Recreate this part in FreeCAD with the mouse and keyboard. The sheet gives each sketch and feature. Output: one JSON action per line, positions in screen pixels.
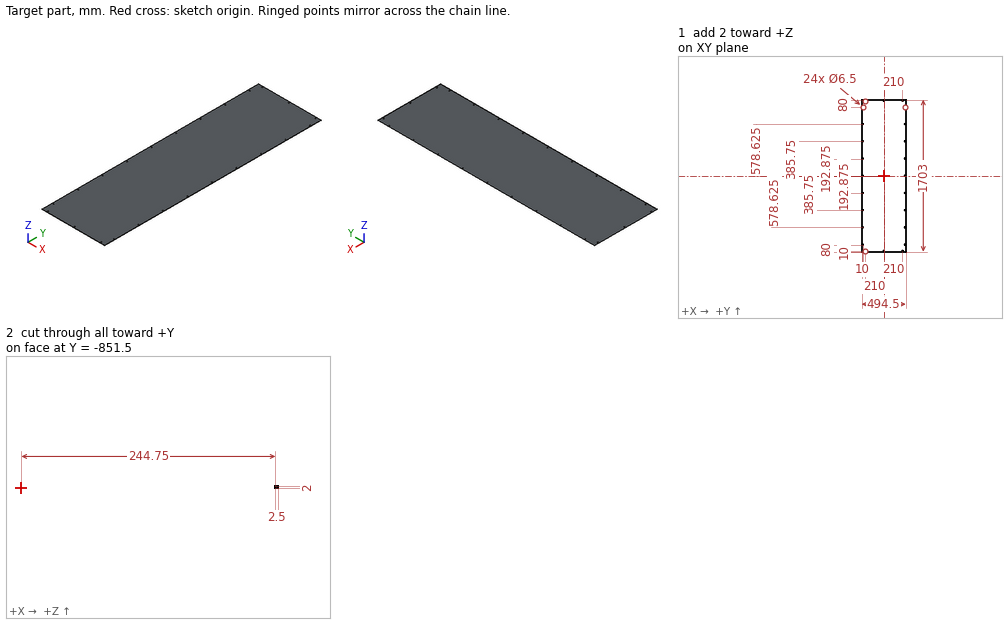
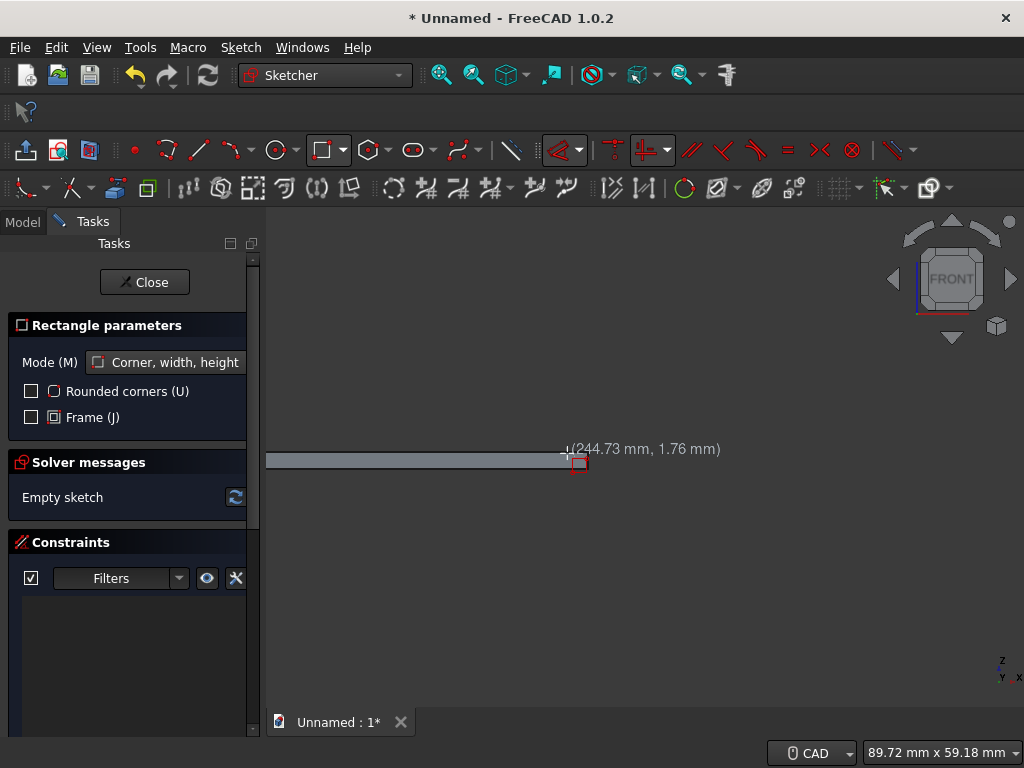
{"action": "left_click", "coordinate": [567, 452]}
{"action": "left_click", "coordinate": [588, 469]}
{"action": "key", "text": "Escape"}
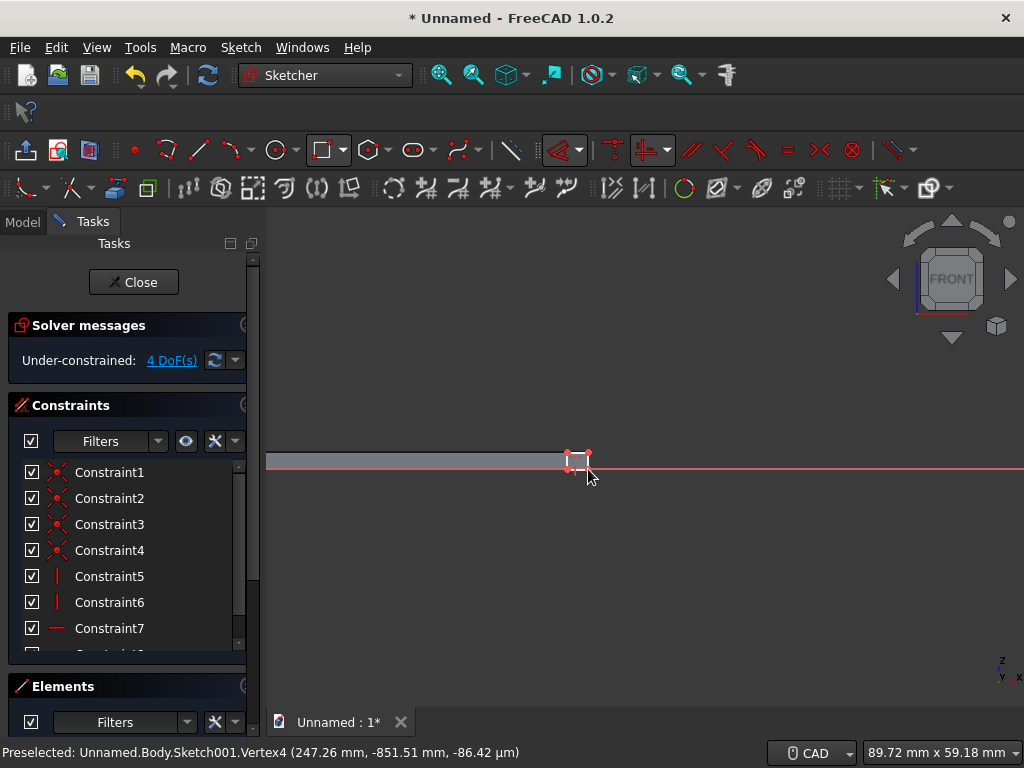
{"action": "left_click", "coordinate": [567, 470]}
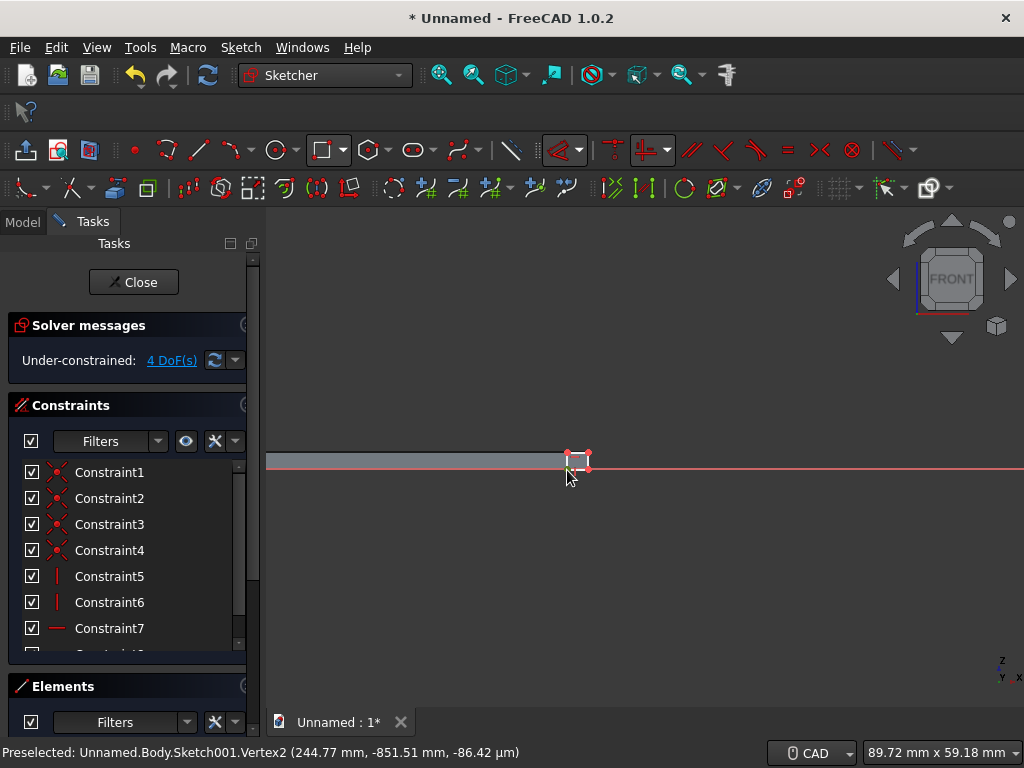
{"action": "left_click", "coordinate": [334, 469]}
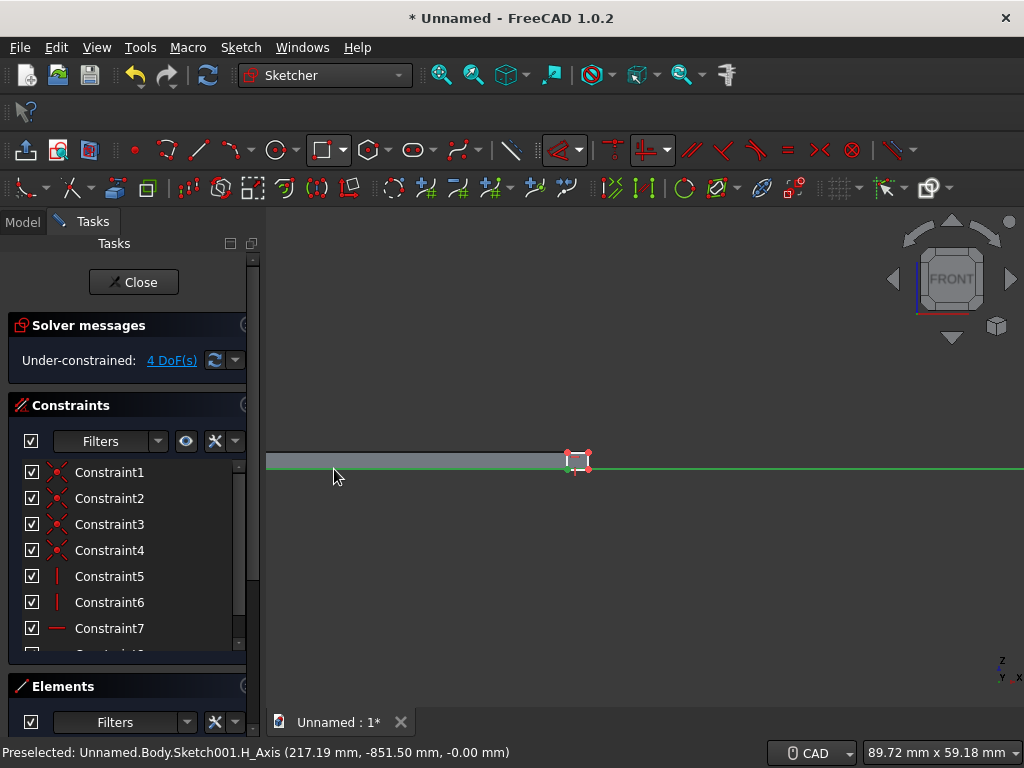
{"action": "left_click", "coordinate": [614, 150]}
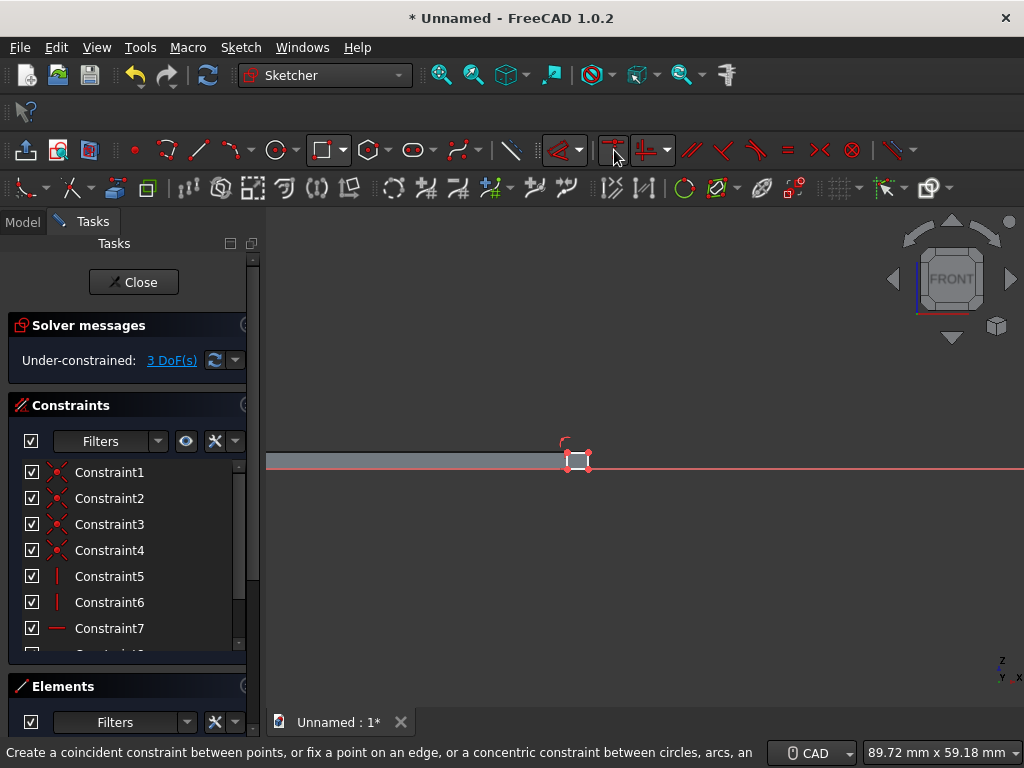
{"action": "scroll", "coordinate": [567, 461], "scroll_direction": "up", "scroll_amount": 5}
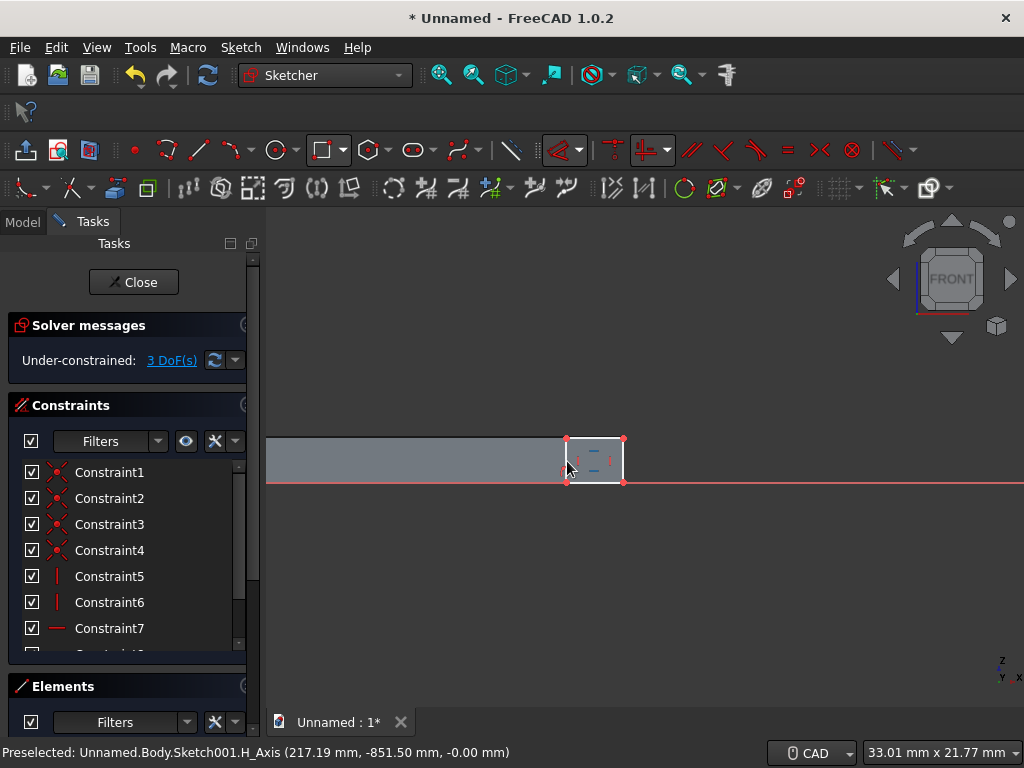
{"action": "left_click", "coordinate": [566, 460]}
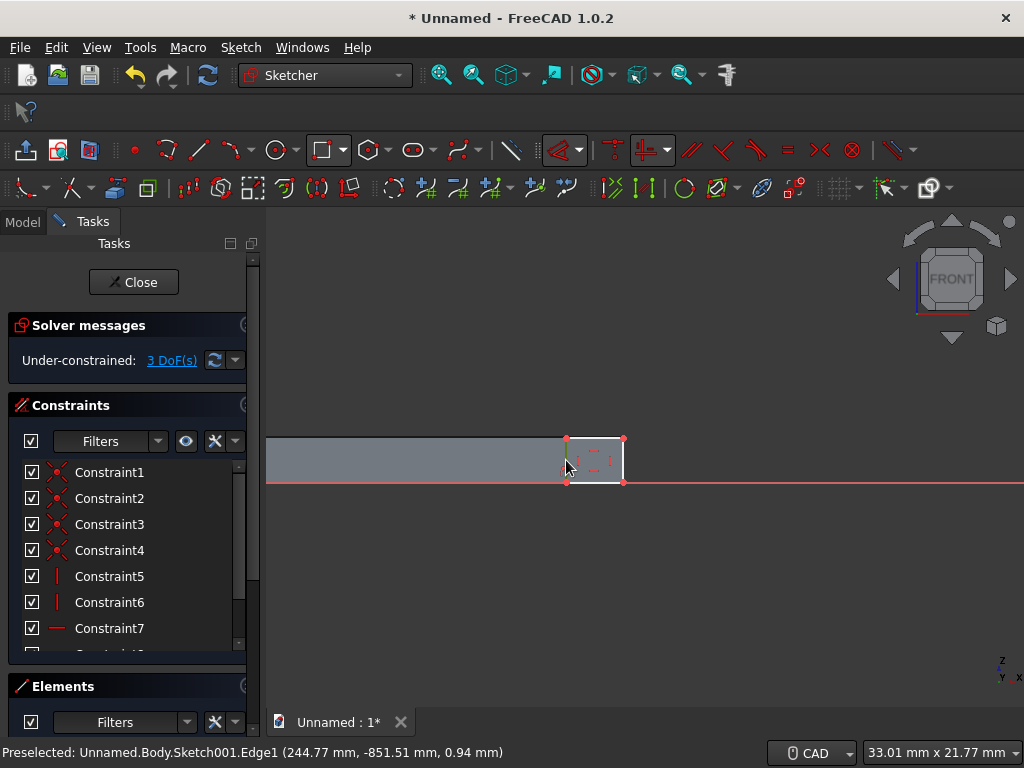
{"action": "left_click", "coordinate": [582, 150]}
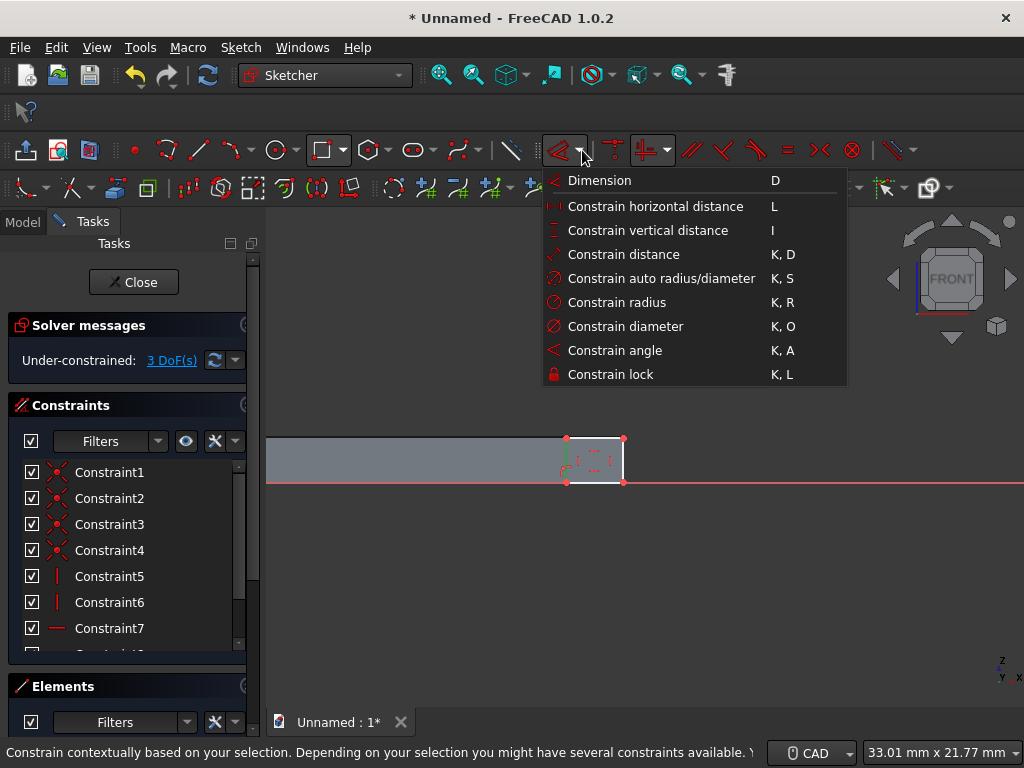
{"action": "left_click", "coordinate": [695, 230]}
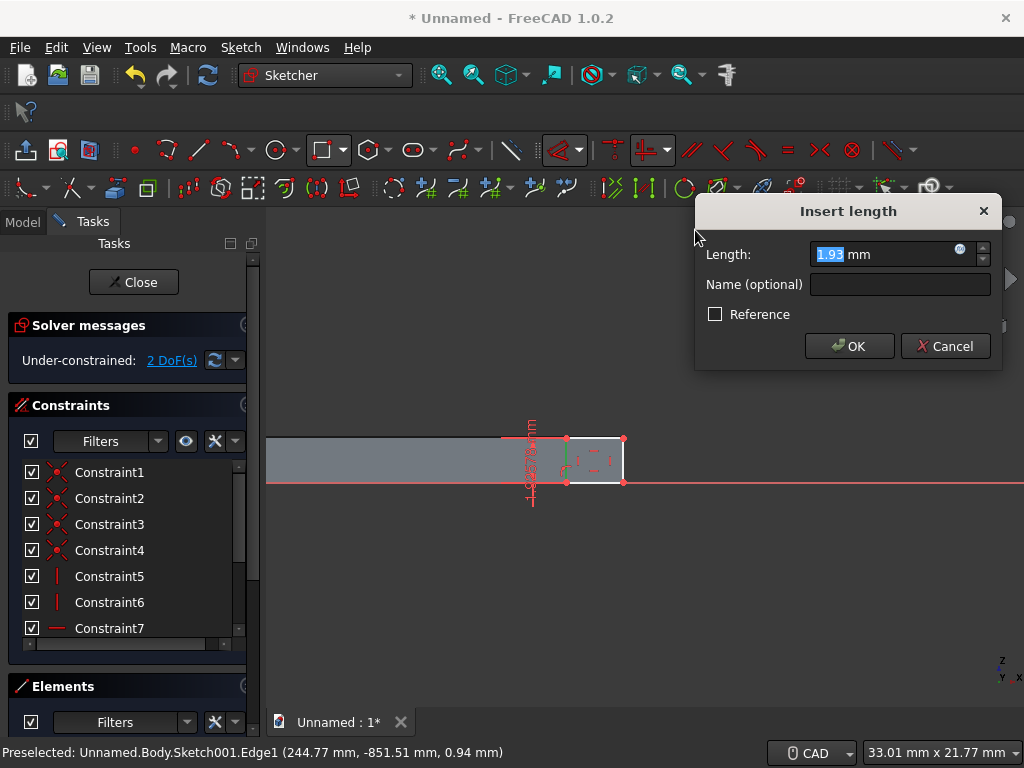
{"action": "type", "text": "2"}
{"action": "key", "text": "Return"}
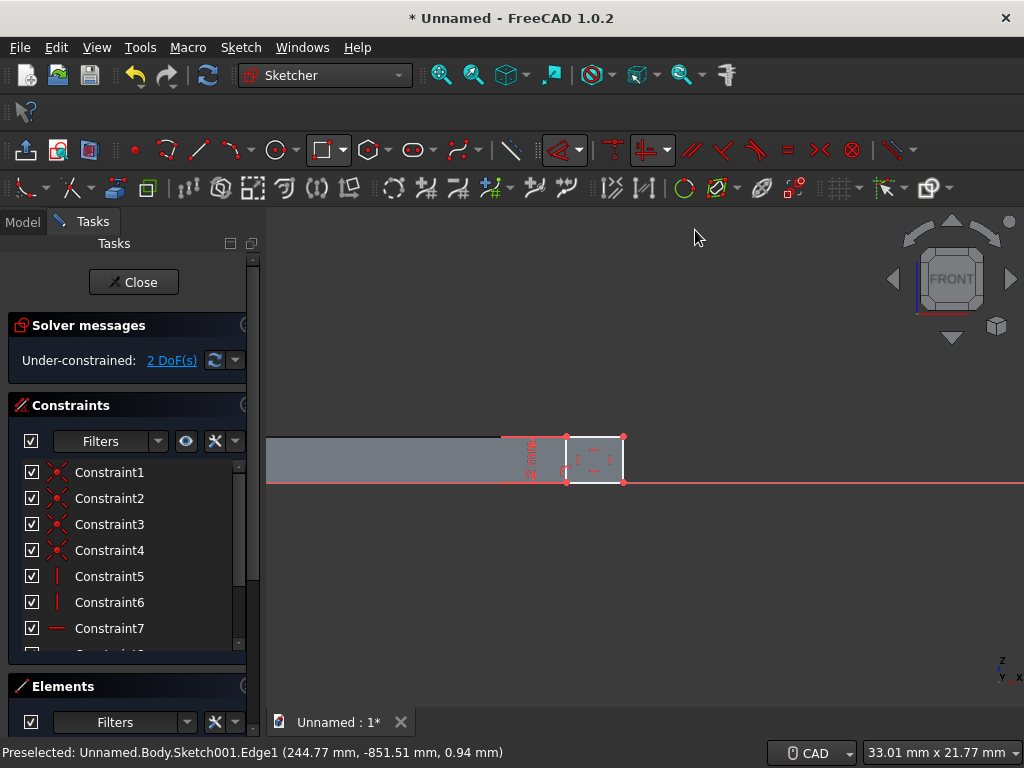
{"action": "left_click", "coordinate": [583, 483]}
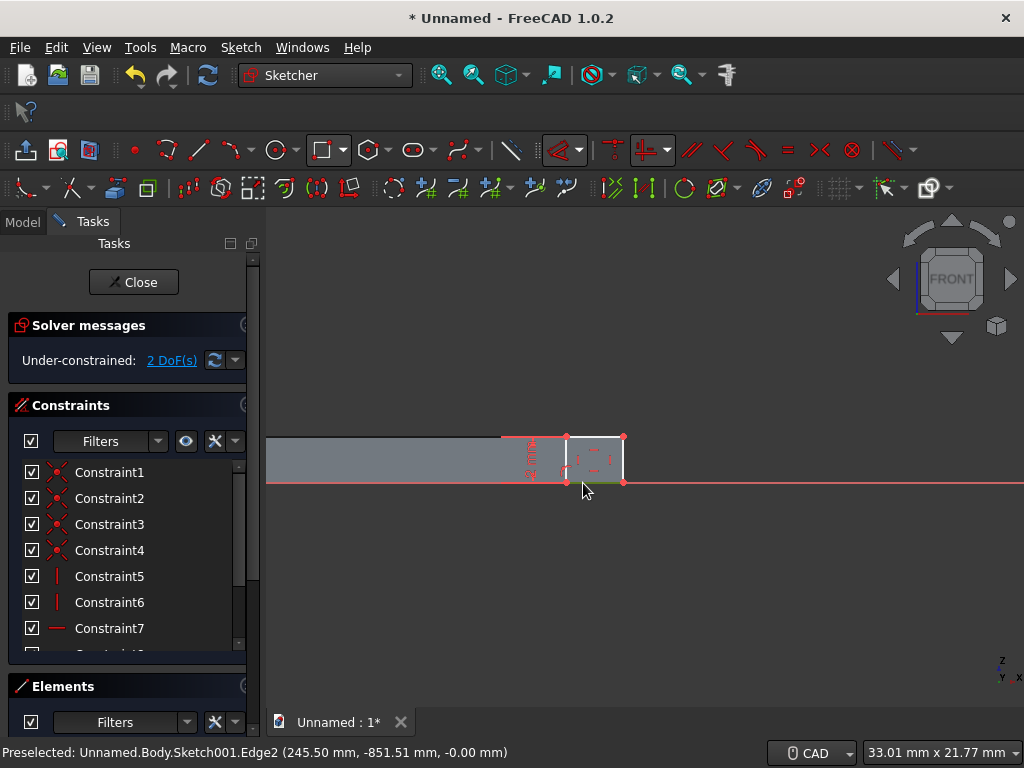
{"action": "left_click", "coordinate": [582, 150]}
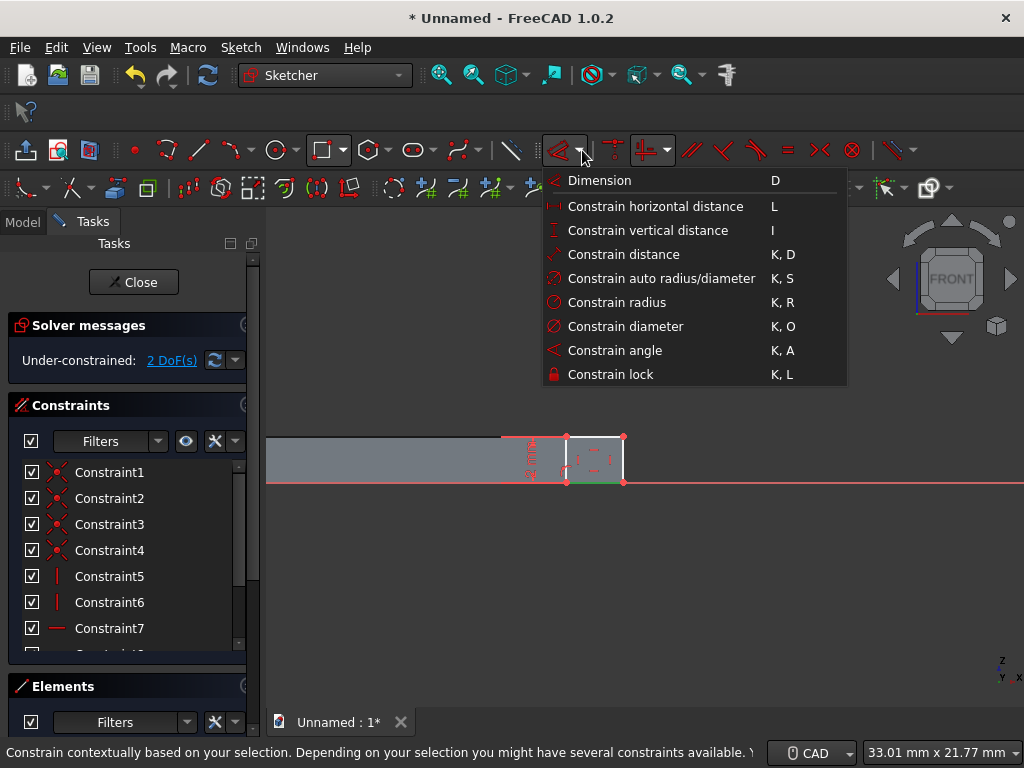
{"action": "left_click", "coordinate": [695, 206]}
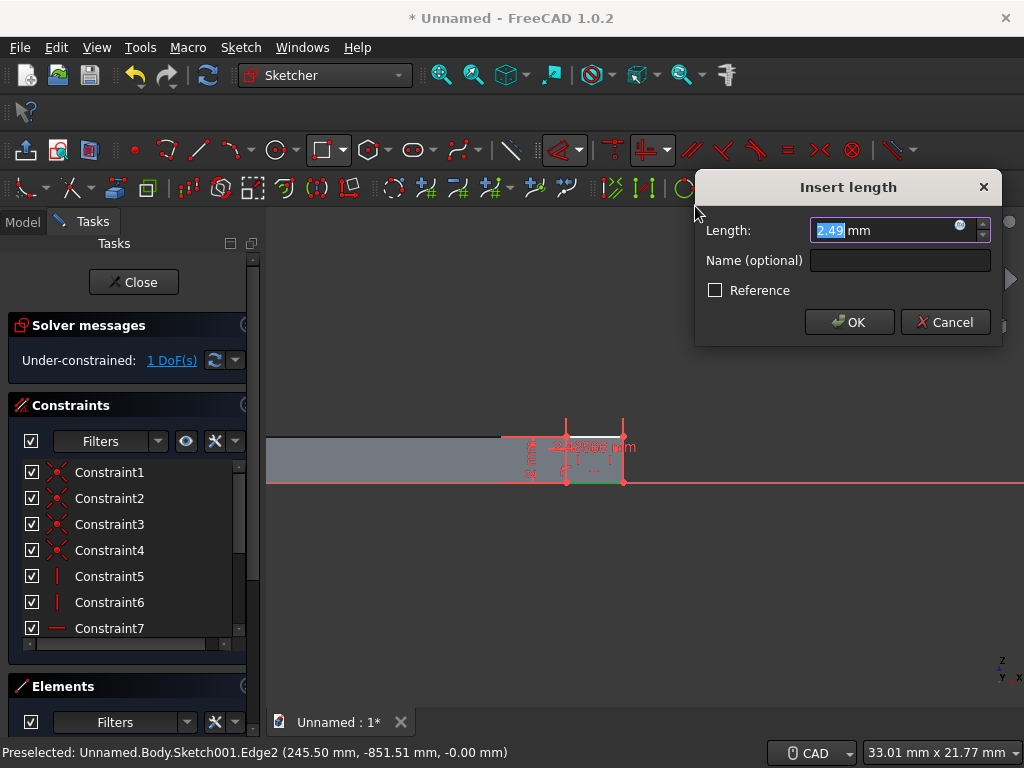
{"action": "type", "text": "2.5"}
{"action": "key", "text": "Return"}